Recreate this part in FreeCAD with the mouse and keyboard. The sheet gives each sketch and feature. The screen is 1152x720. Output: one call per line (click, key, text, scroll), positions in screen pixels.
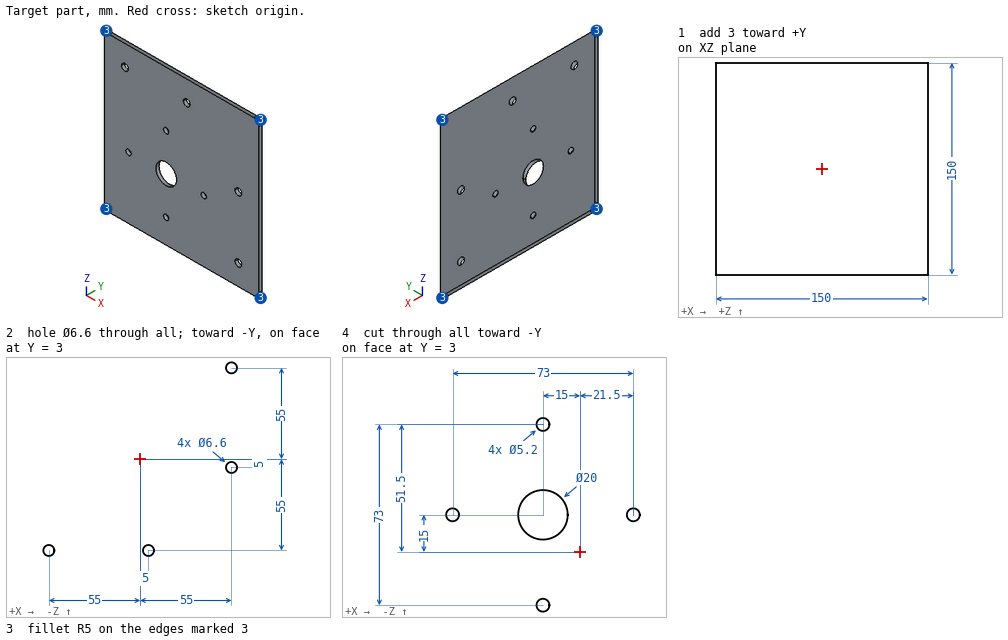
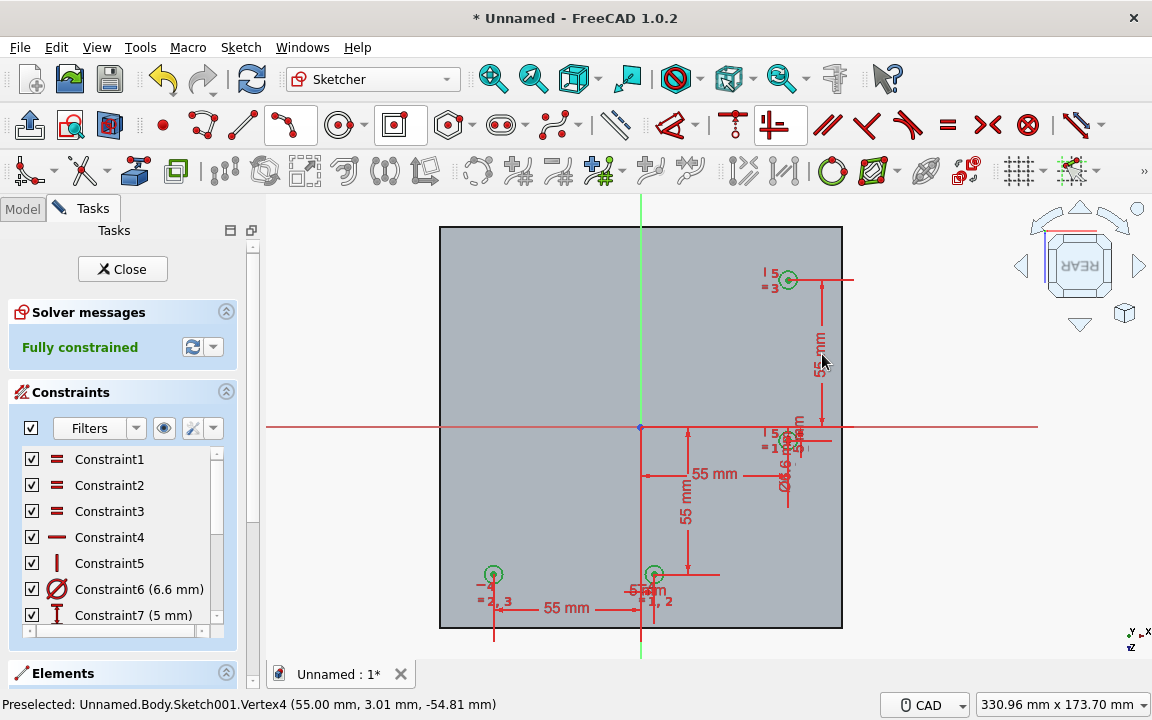
click(123, 269)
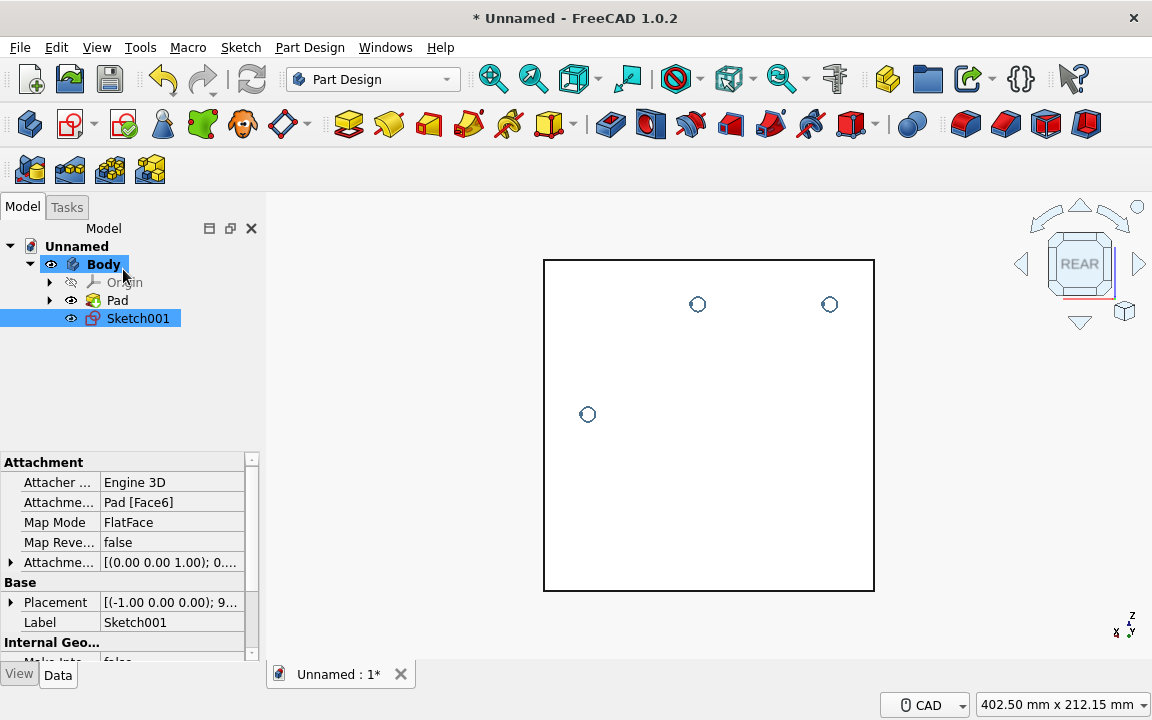
click(652, 124)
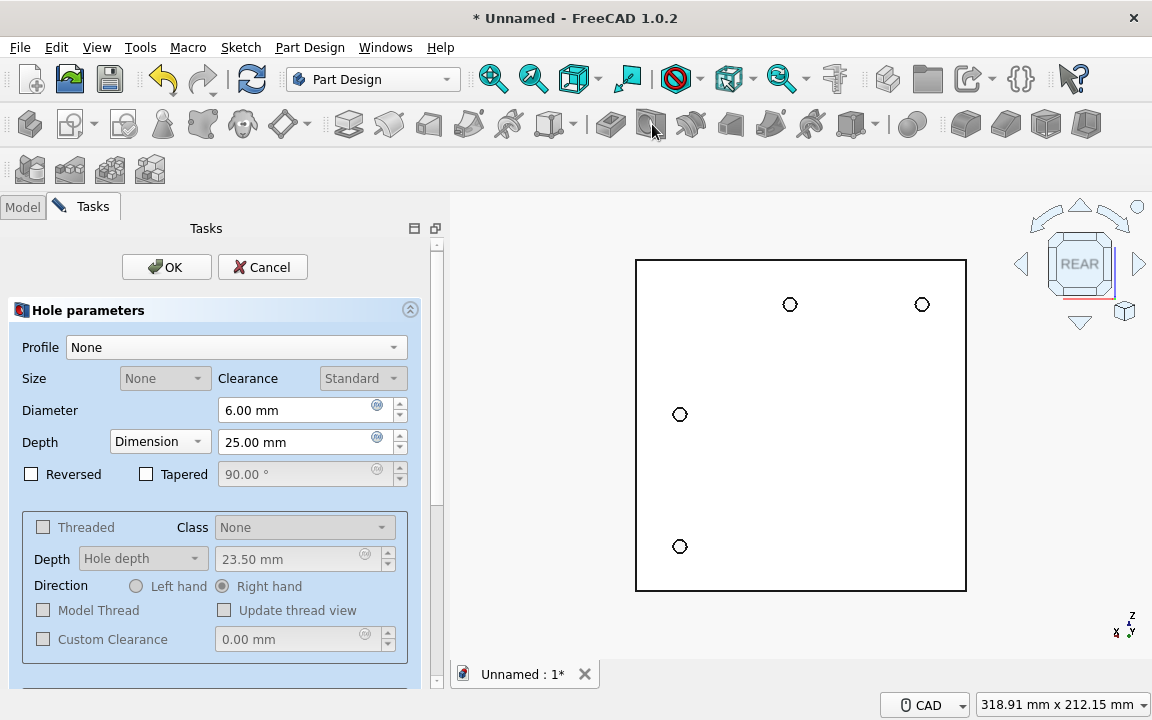
triple_click(305, 410)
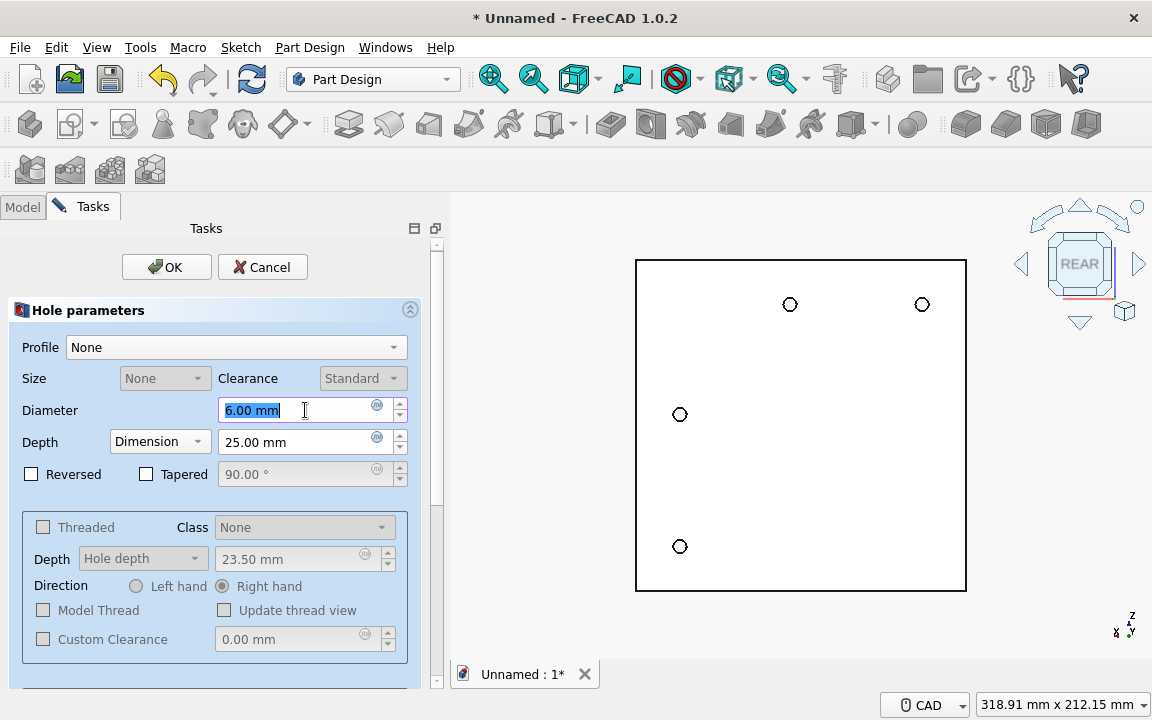
text(6.6)
key(Tab)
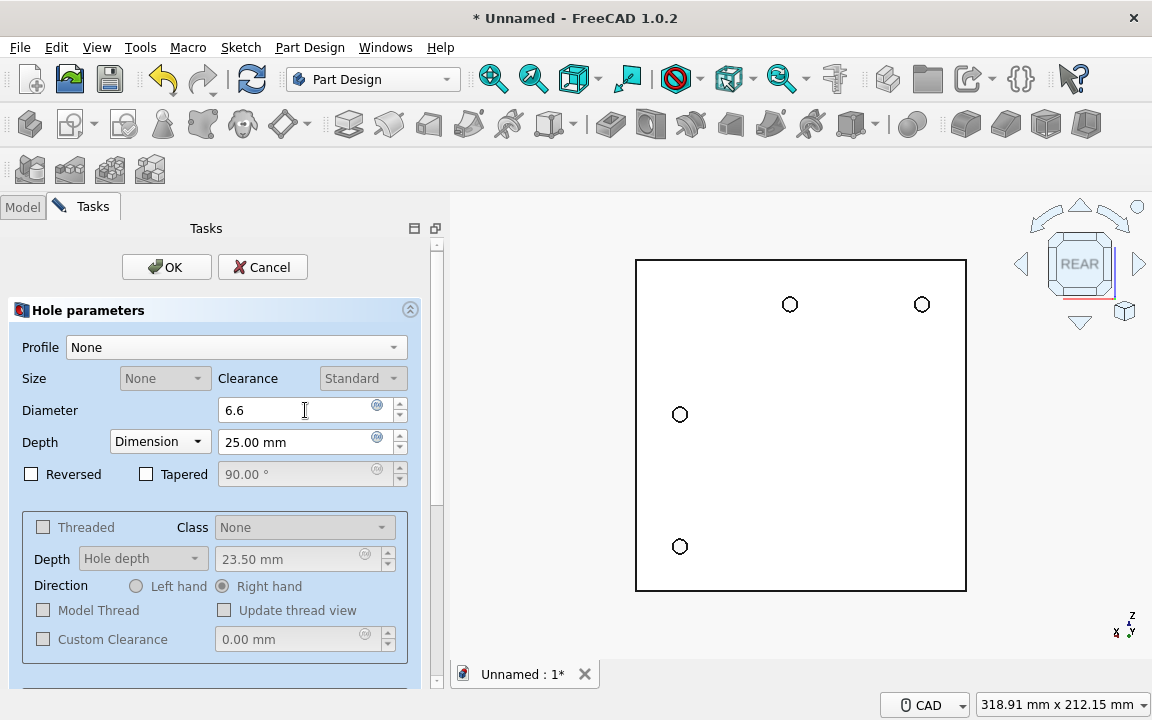
click(161, 442)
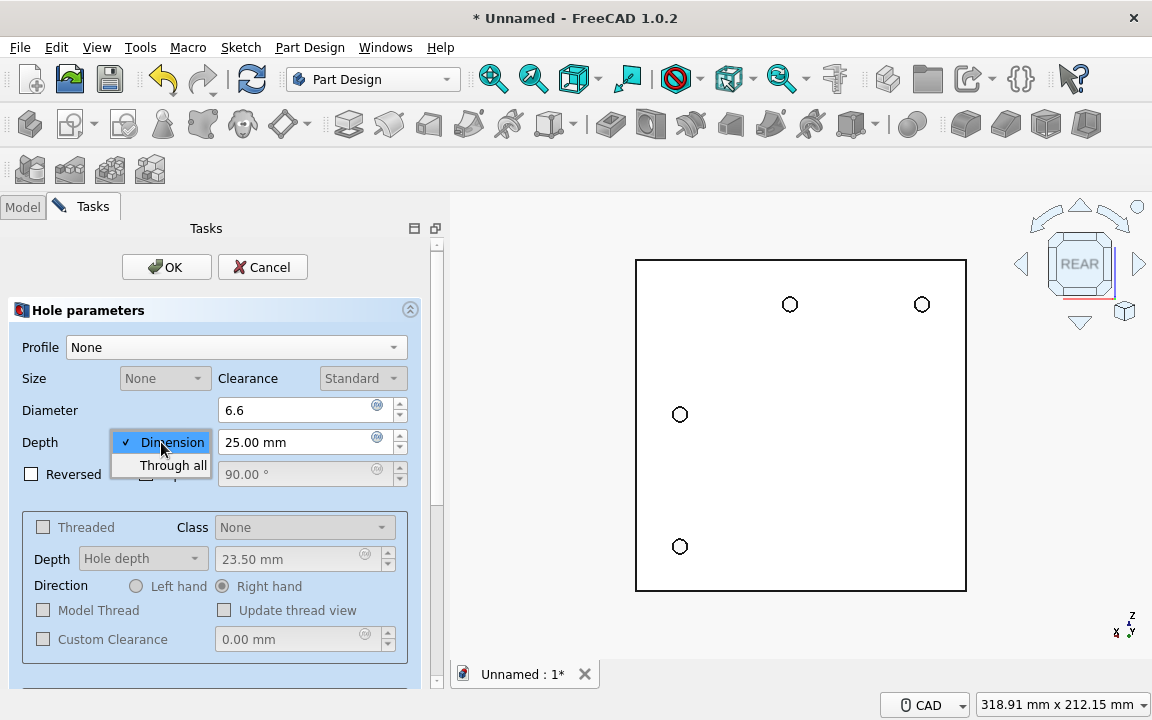
click(160, 466)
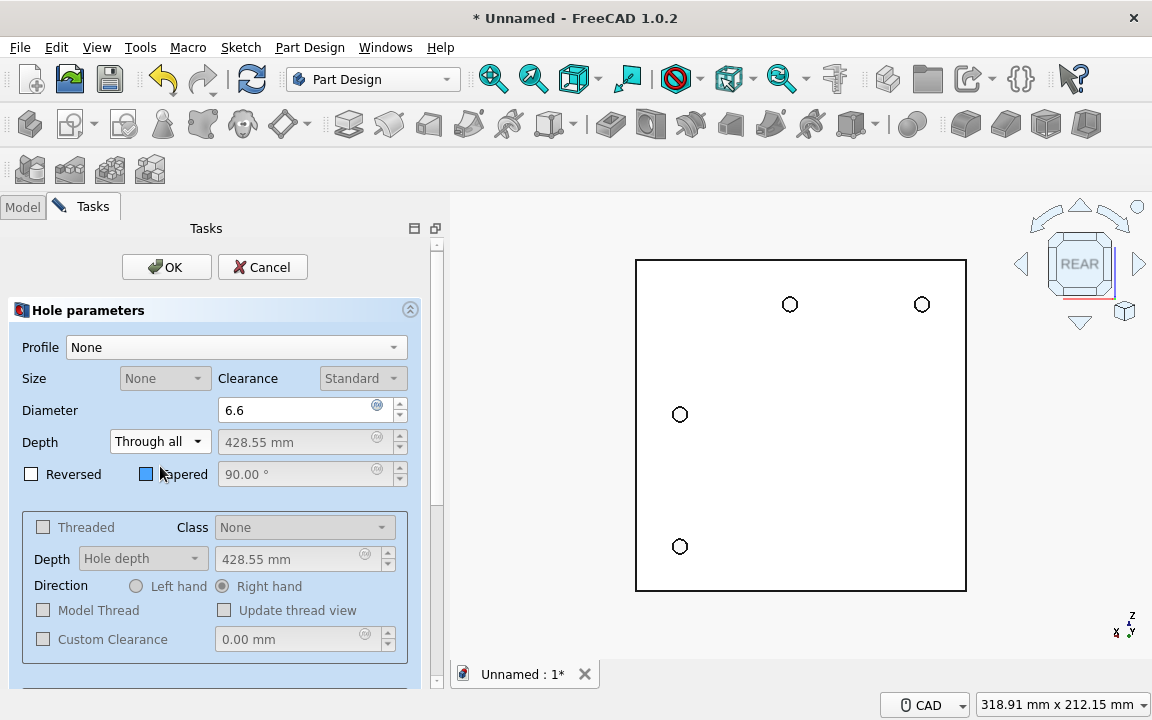
click(167, 267)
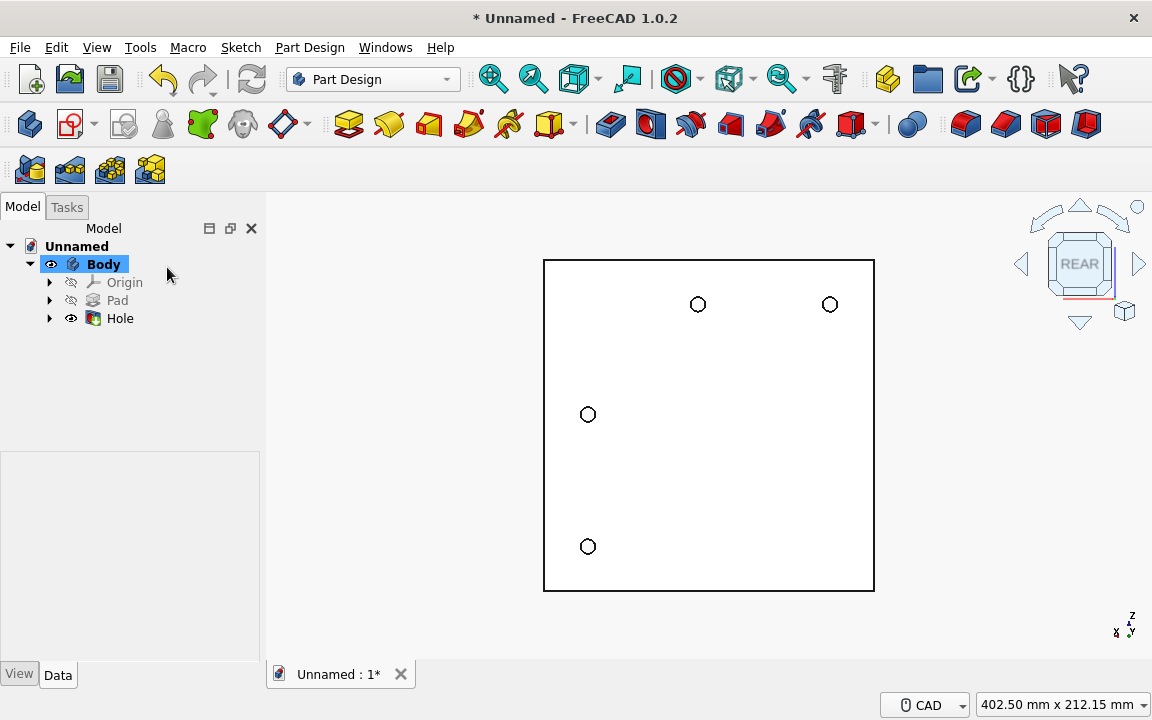
scroll(544, 259, up, 10)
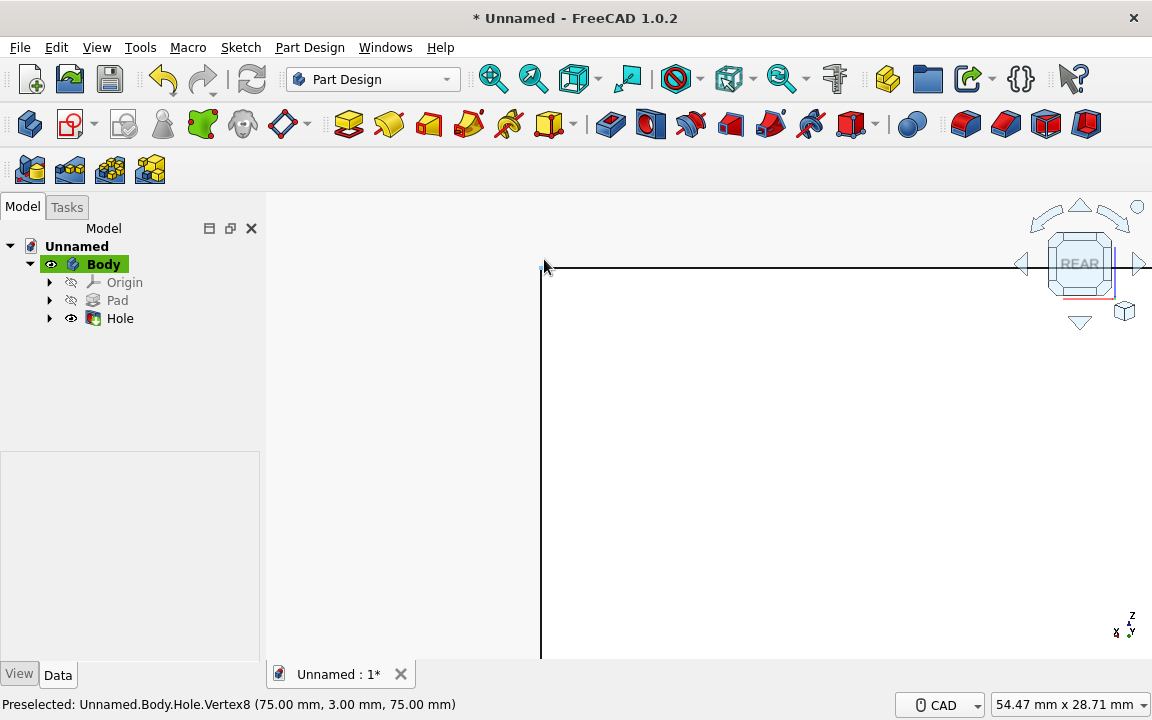
click(494, 80)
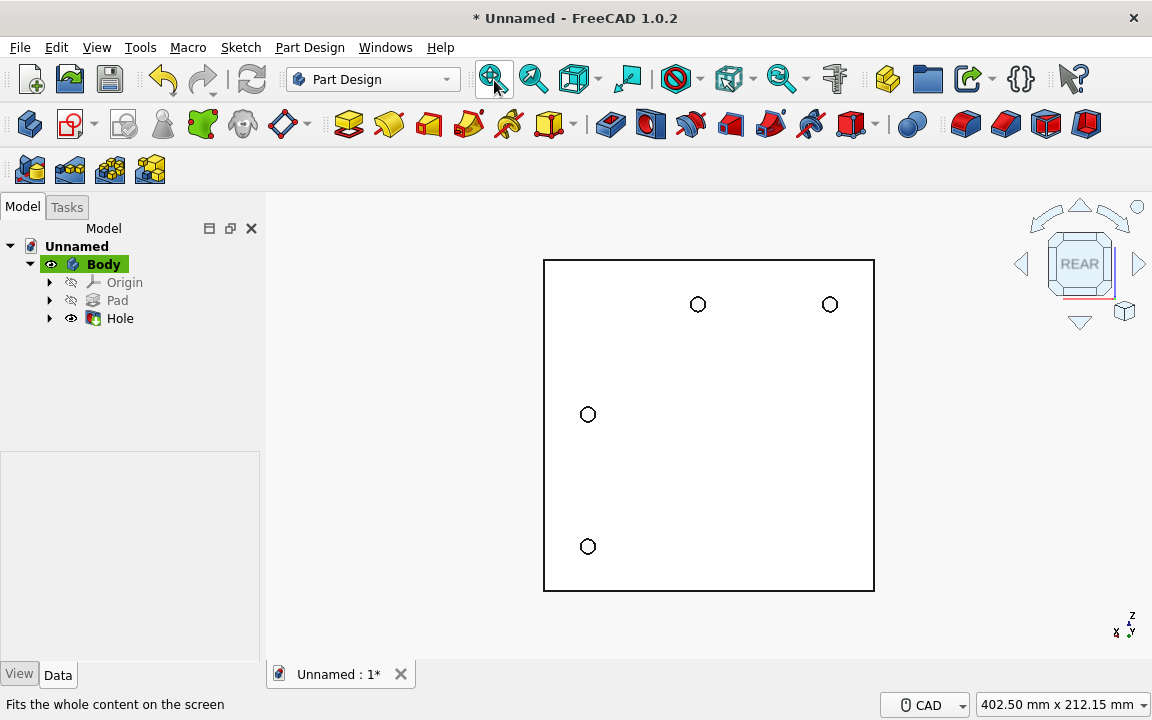
key(0)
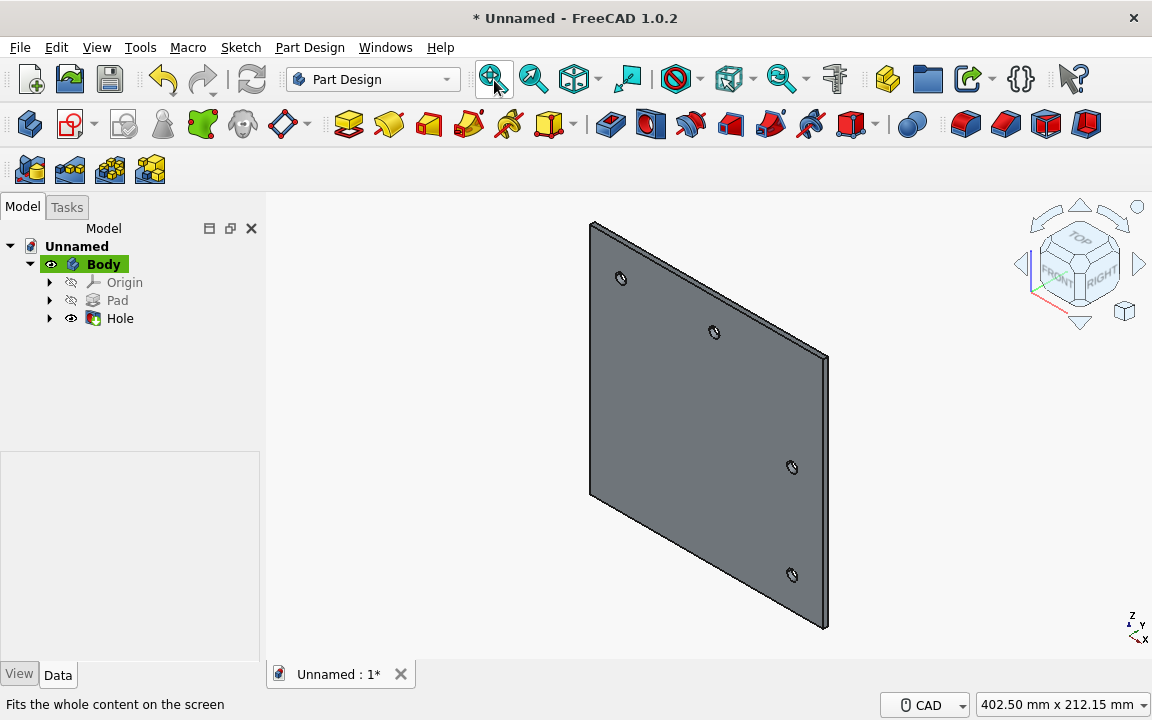
scroll(826, 357, up, 10)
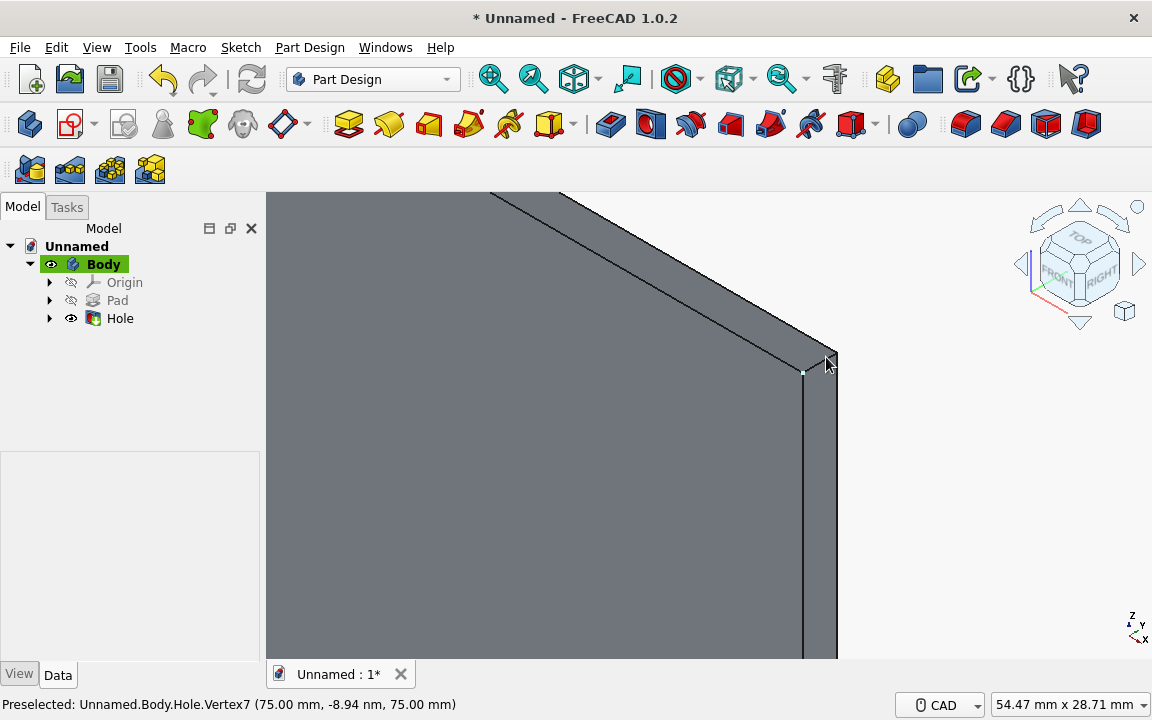
click(820, 362)